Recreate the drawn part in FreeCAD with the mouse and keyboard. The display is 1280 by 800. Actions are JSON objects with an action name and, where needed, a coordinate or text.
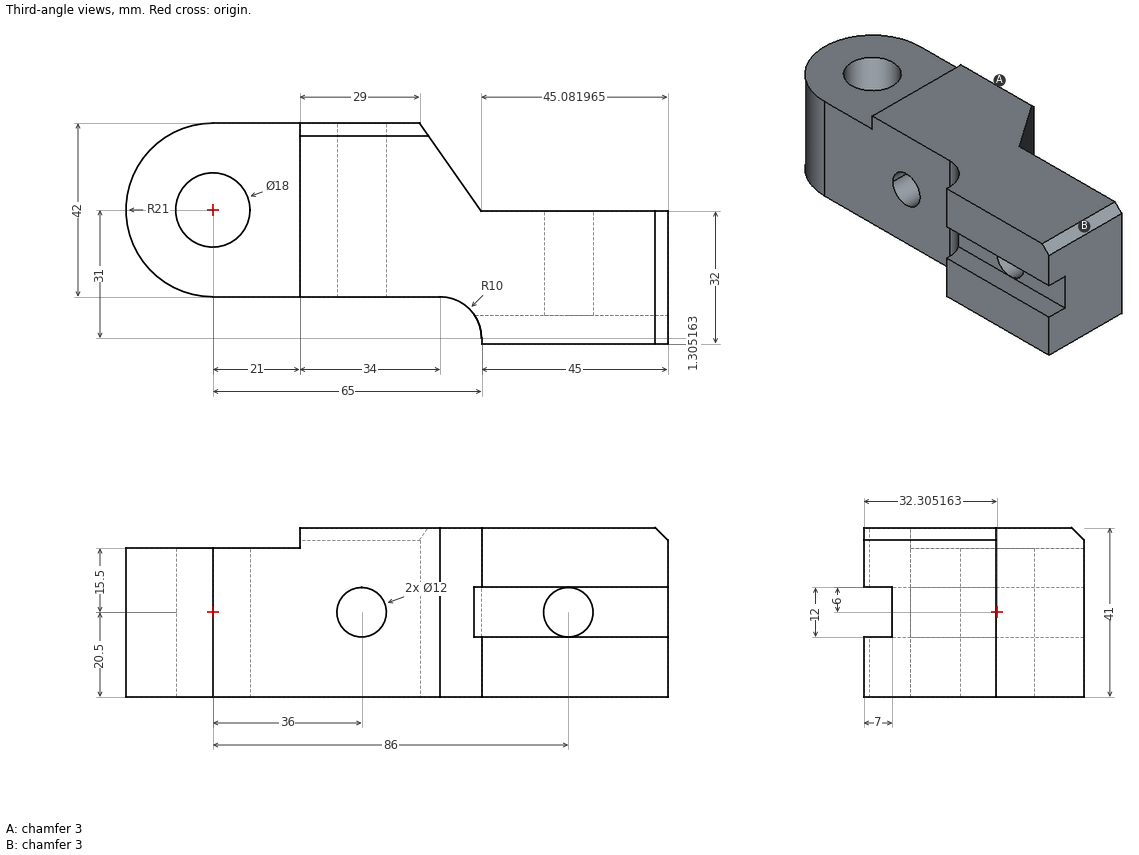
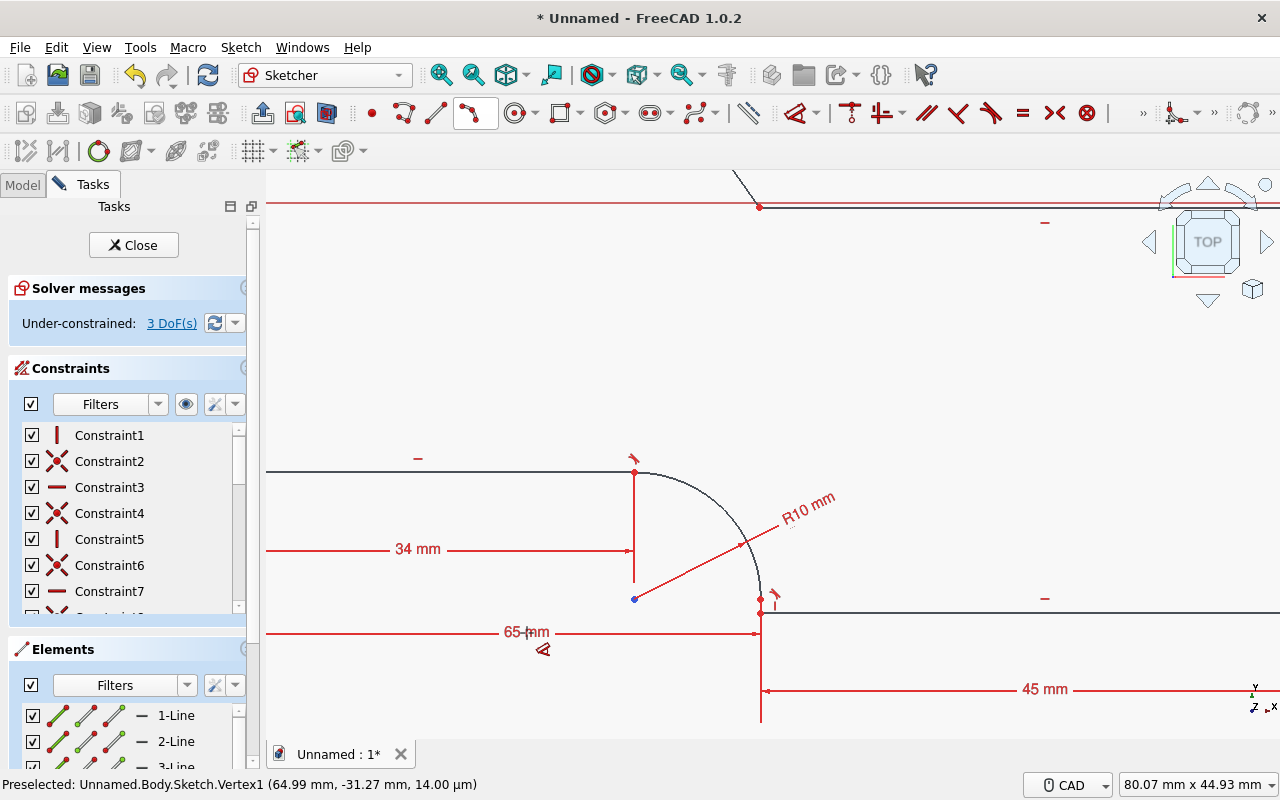
{"action": "left_click", "coordinate": [761, 599]}
{"action": "left_click", "coordinate": [795, 401]}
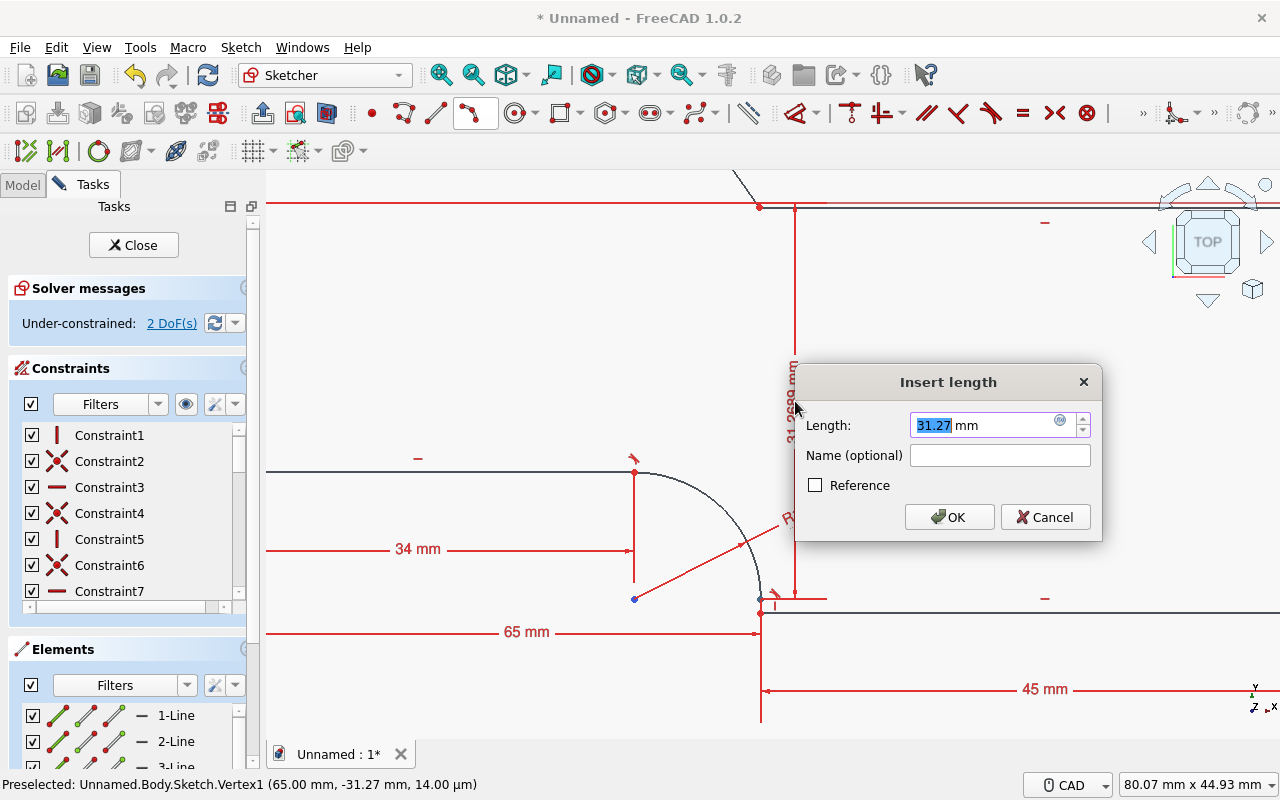
{"action": "type", "text": "31"}
{"action": "key", "text": "Return"}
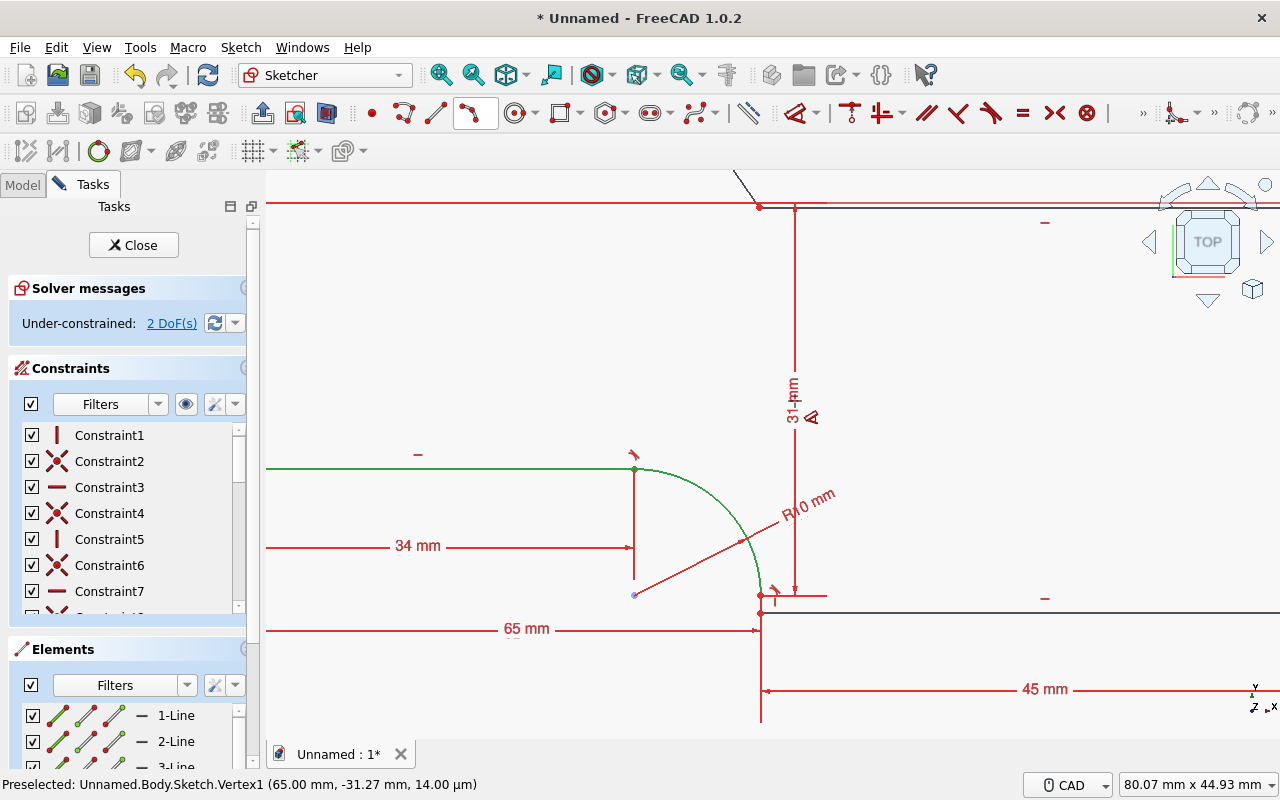
{"action": "scroll", "coordinate": [761, 604], "scroll_direction": "up", "scroll_amount": 5}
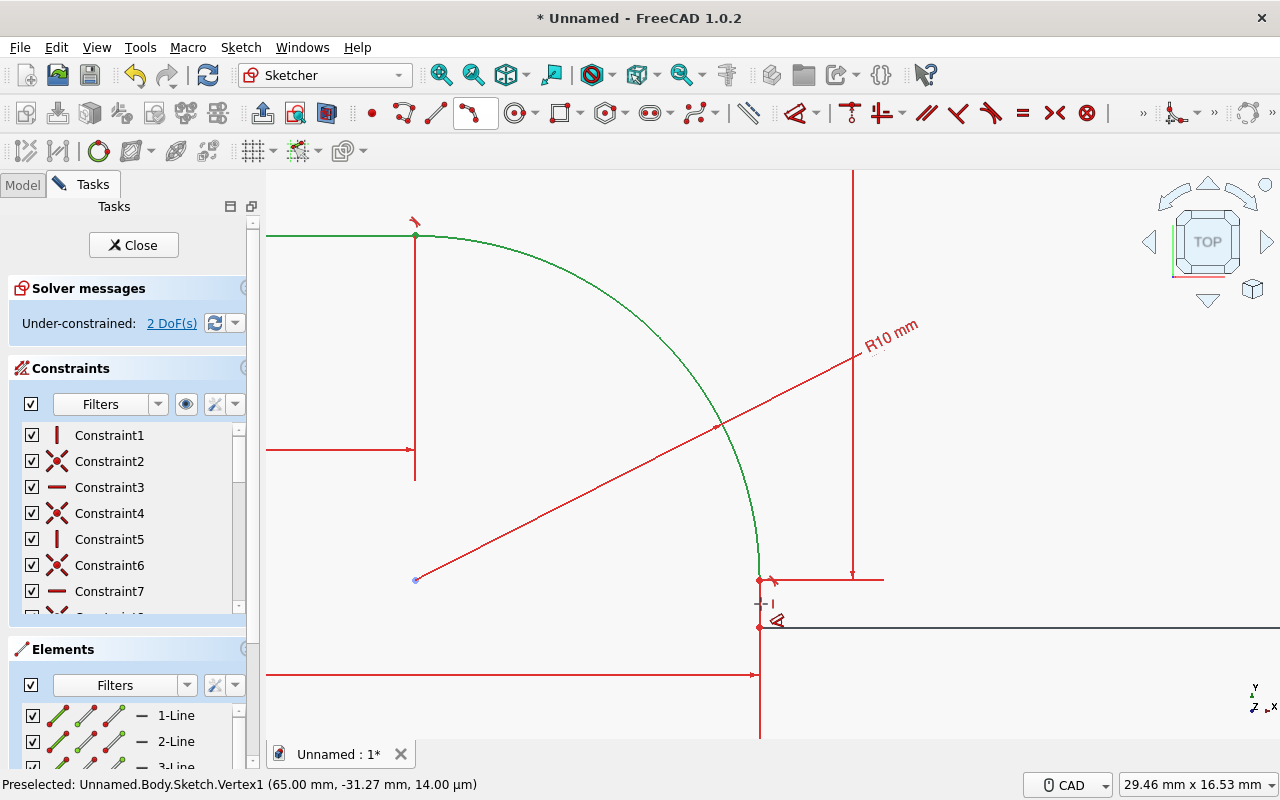
{"action": "left_click", "coordinate": [760, 604]}
{"action": "left_click", "coordinate": [794, 604]}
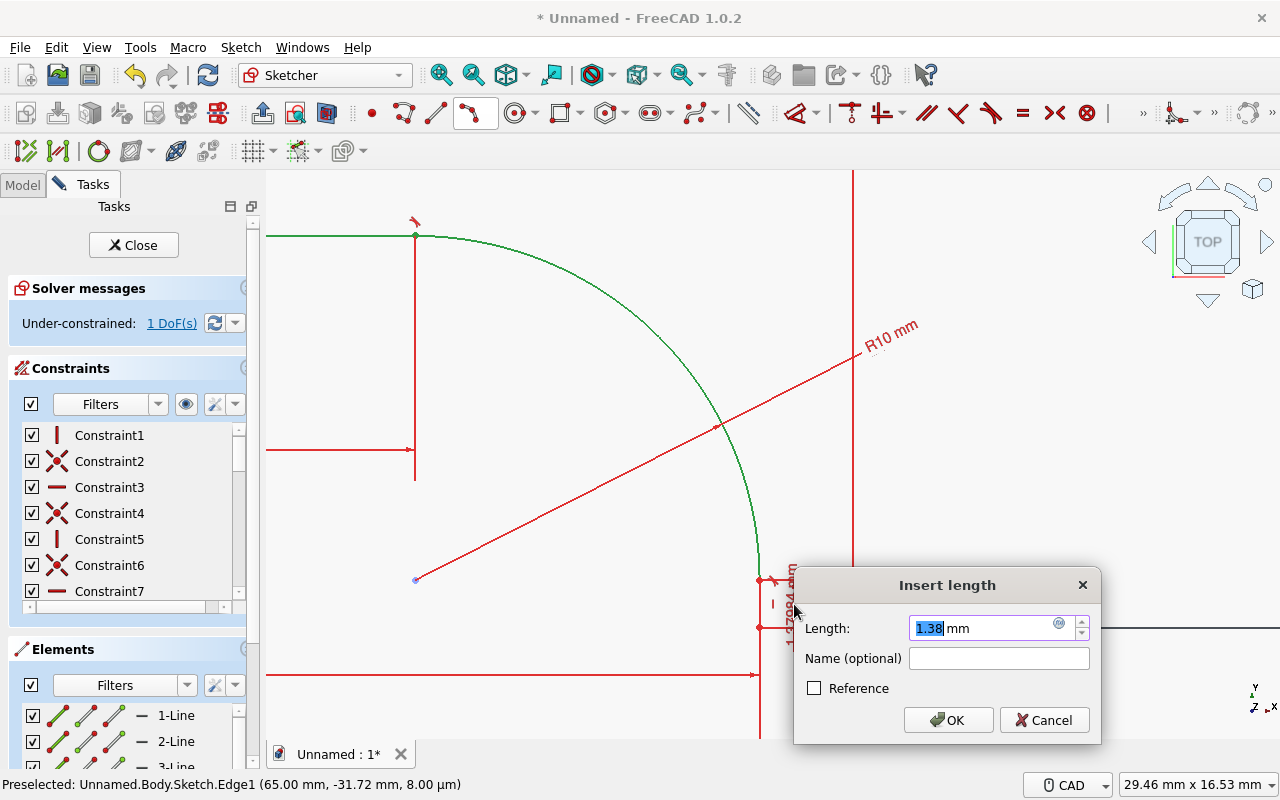
{"action": "type", "text": "1.305163"}
{"action": "key", "text": "Return"}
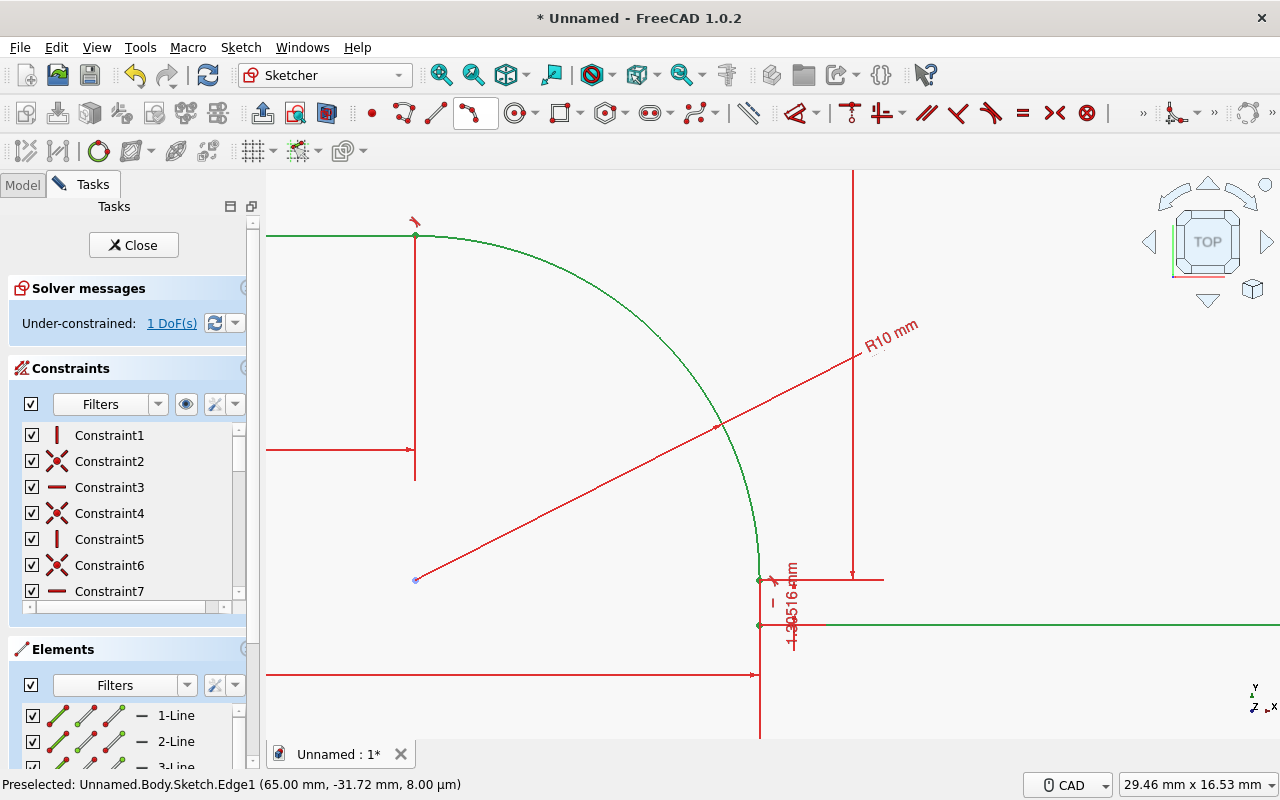
{"action": "scroll", "coordinate": [762, 602], "scroll_direction": "down", "scroll_amount": 9}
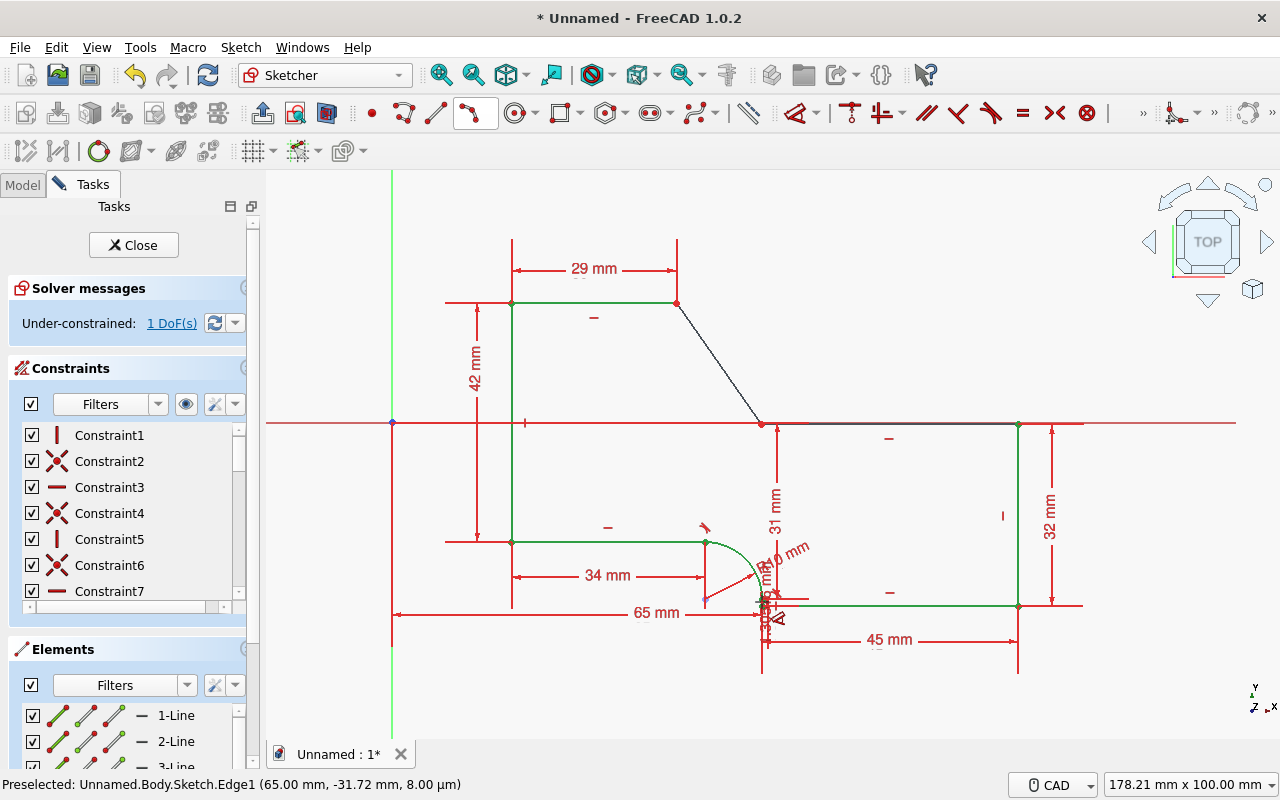
{"action": "scroll", "coordinate": [941, 424], "scroll_direction": "up", "scroll_amount": 11}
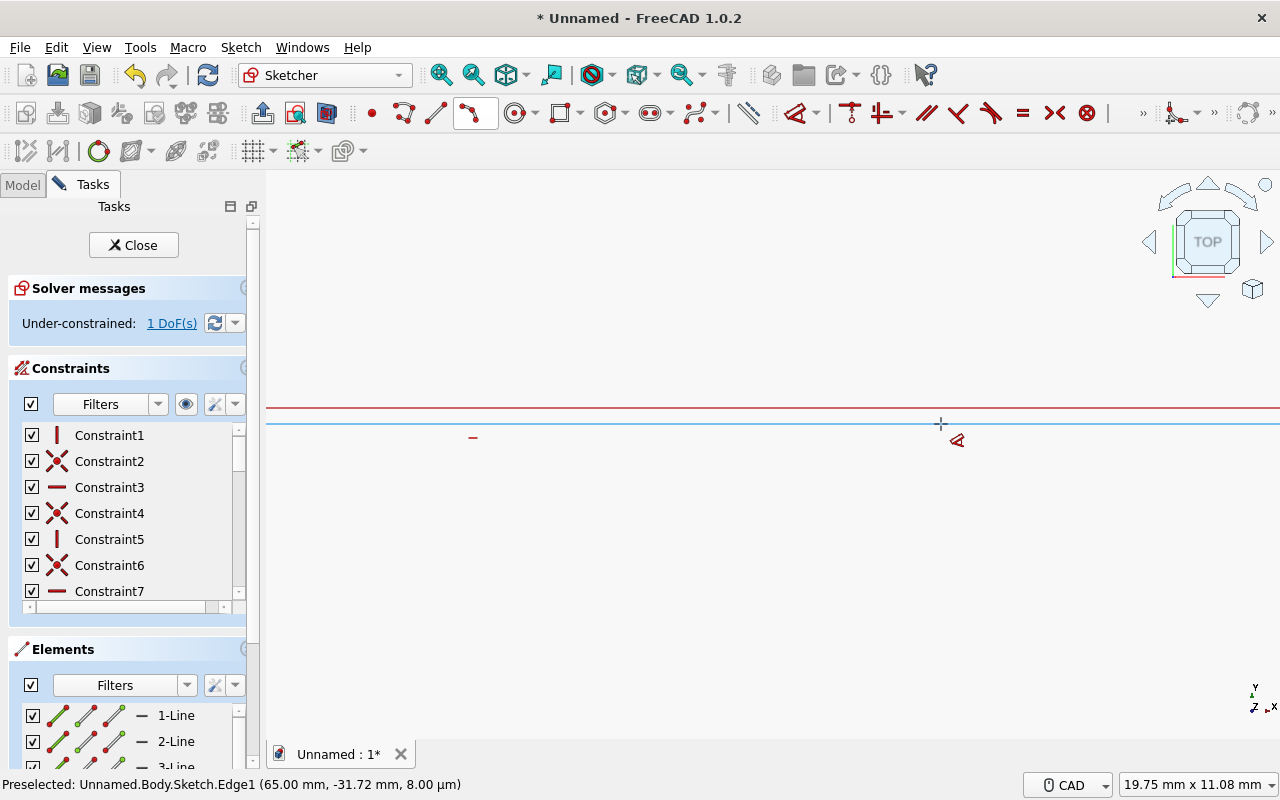
{"action": "left_click", "coordinate": [936, 424]}
{"action": "left_click", "coordinate": [704, 390]}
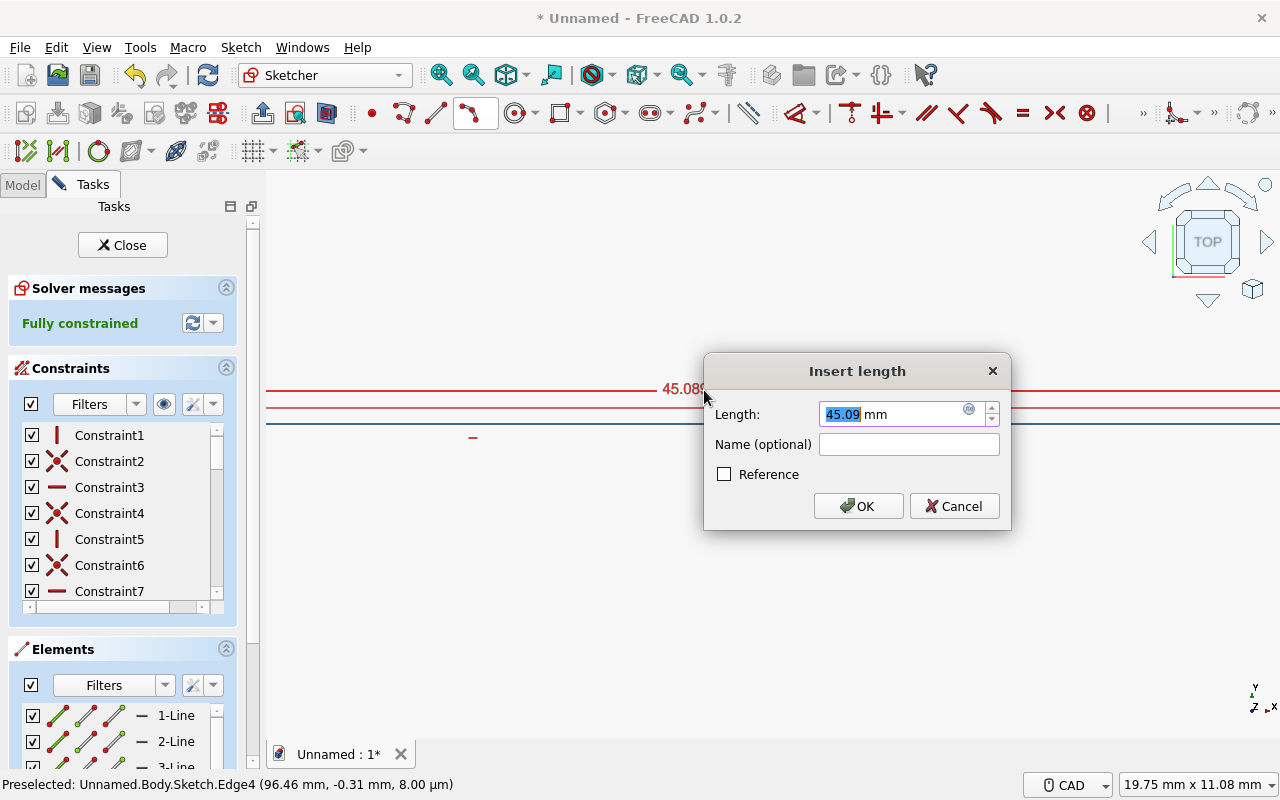
{"action": "type", "text": "45.081965"}
{"action": "key", "text": "Return"}
{"action": "key", "text": "Escape"}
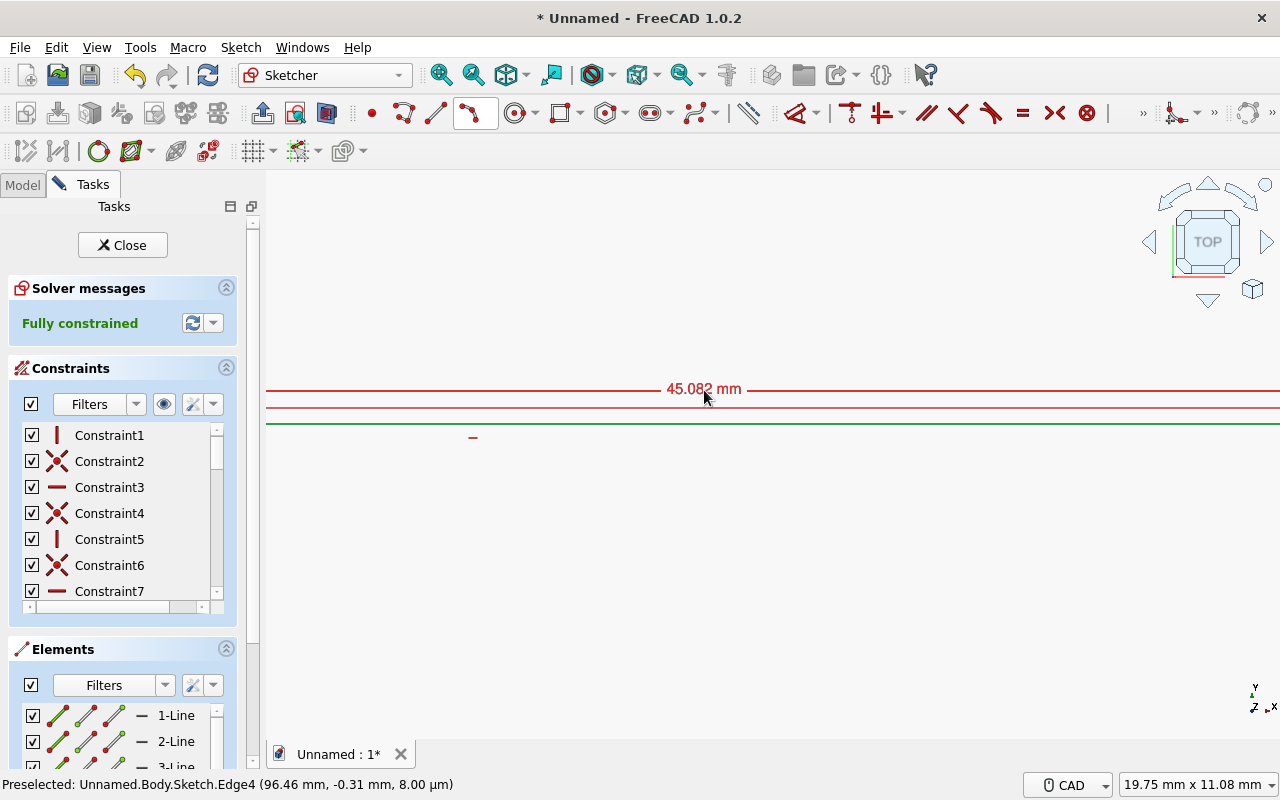
{"action": "left_click", "coordinate": [123, 245]}